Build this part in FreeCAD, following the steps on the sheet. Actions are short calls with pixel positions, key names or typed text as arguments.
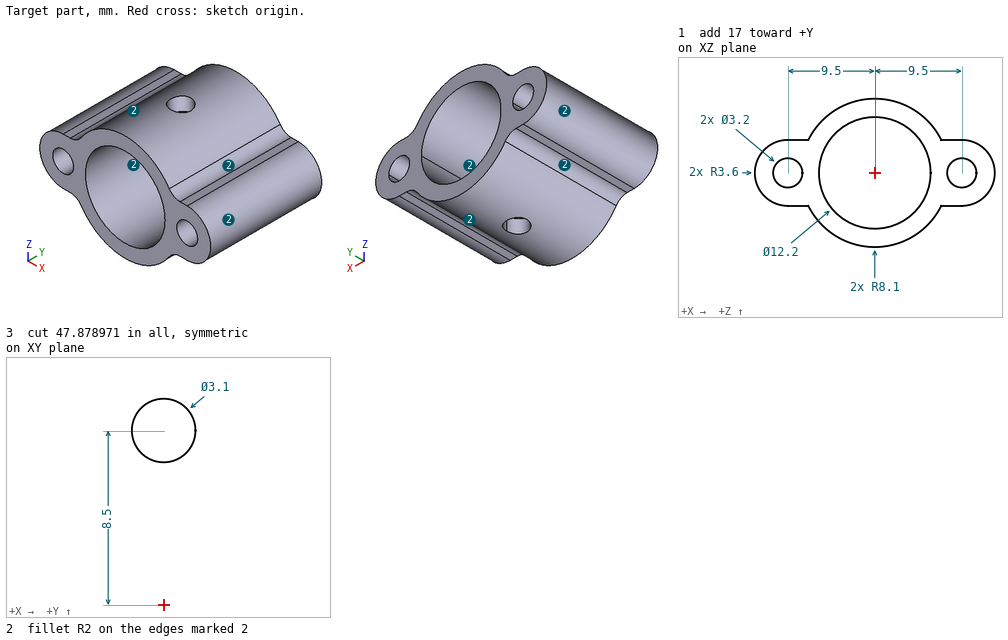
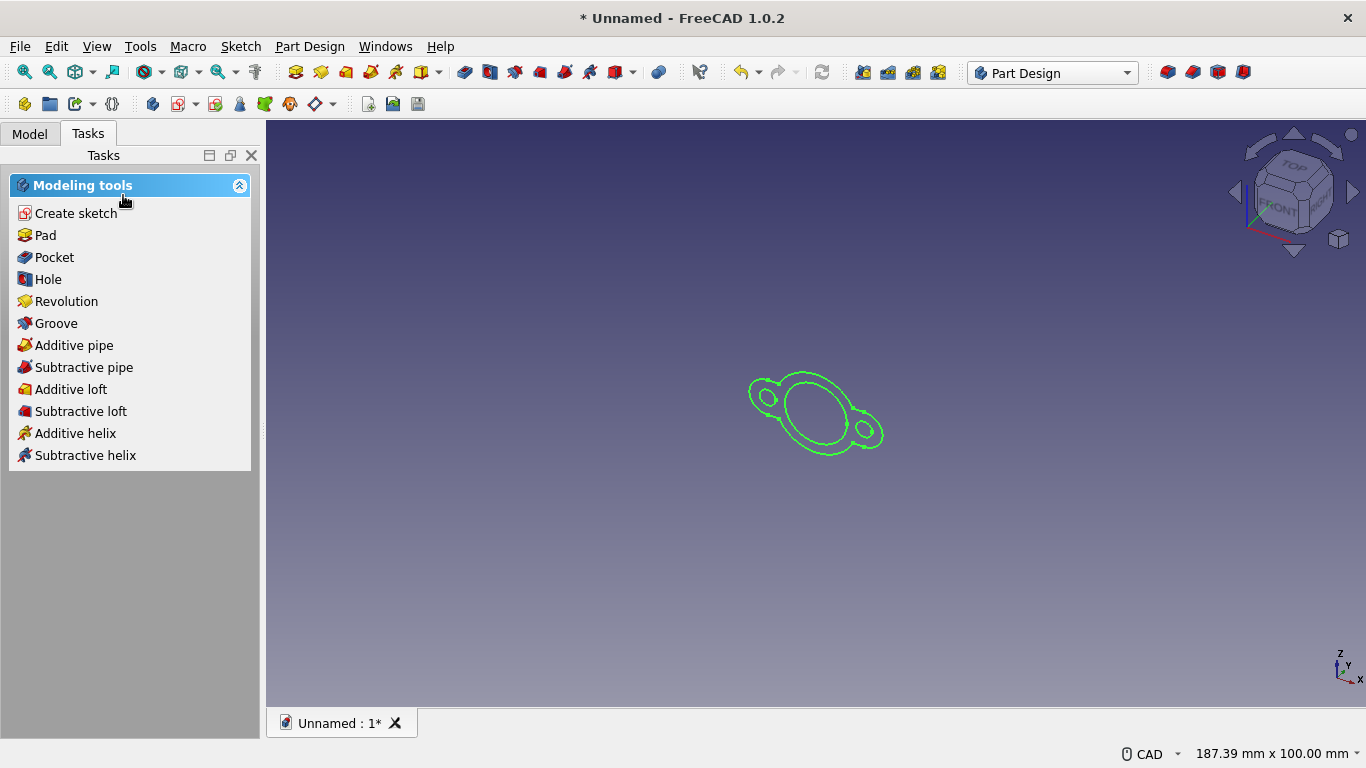
click(296, 72)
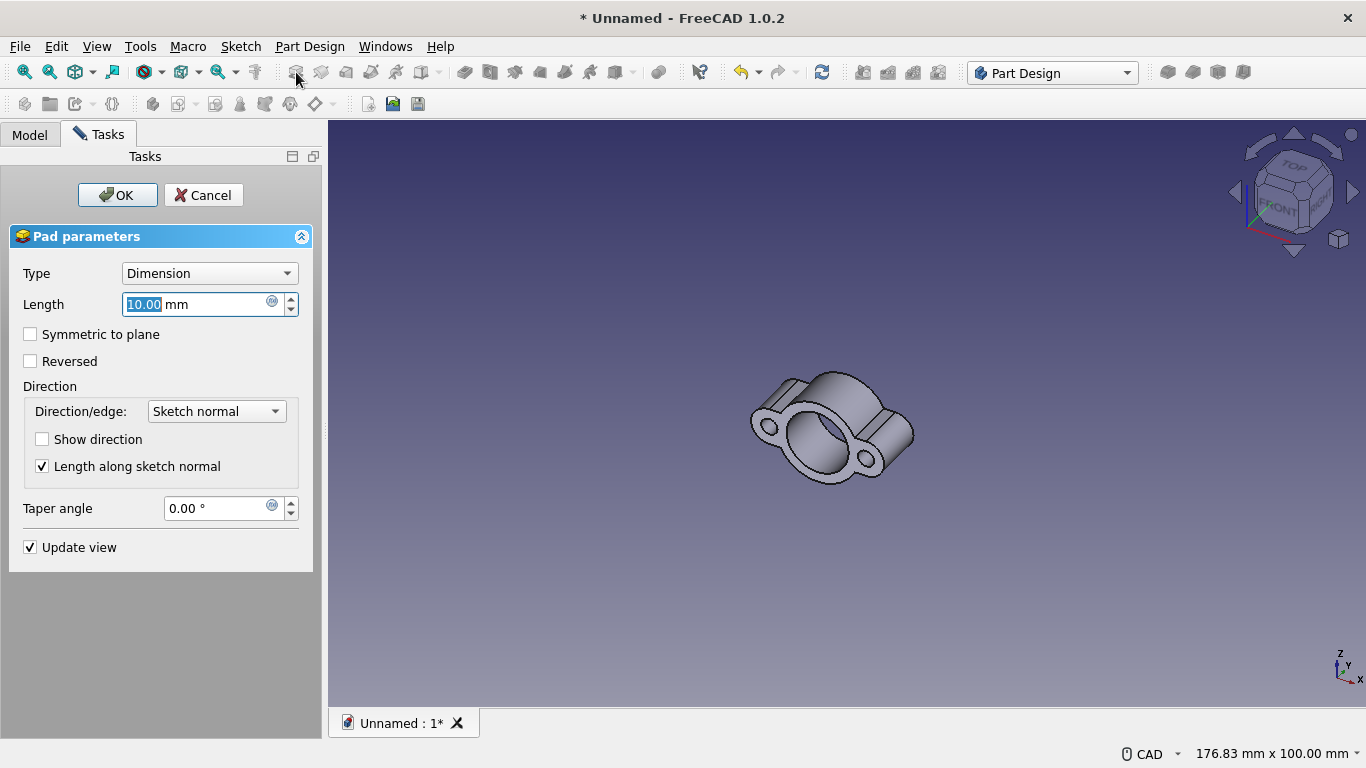
text(17)
key(Tab)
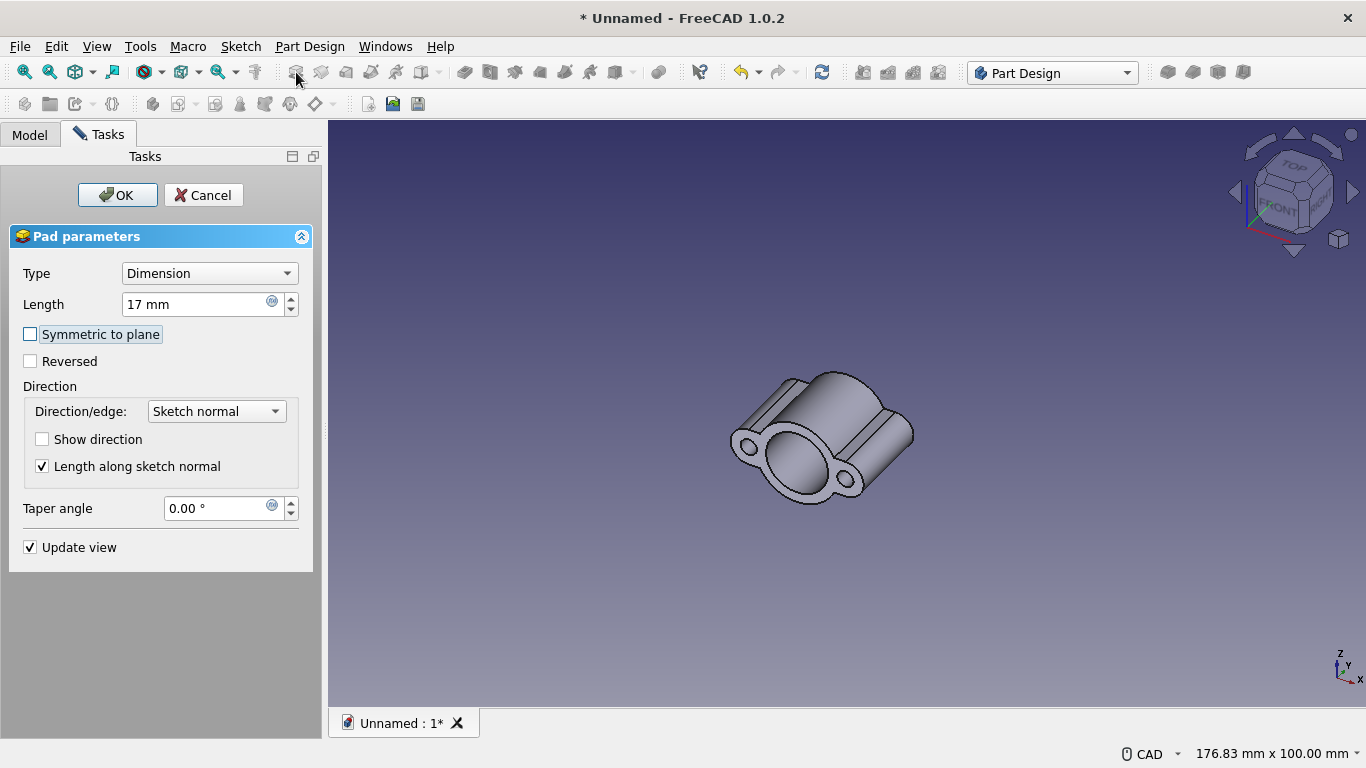
click(31, 361)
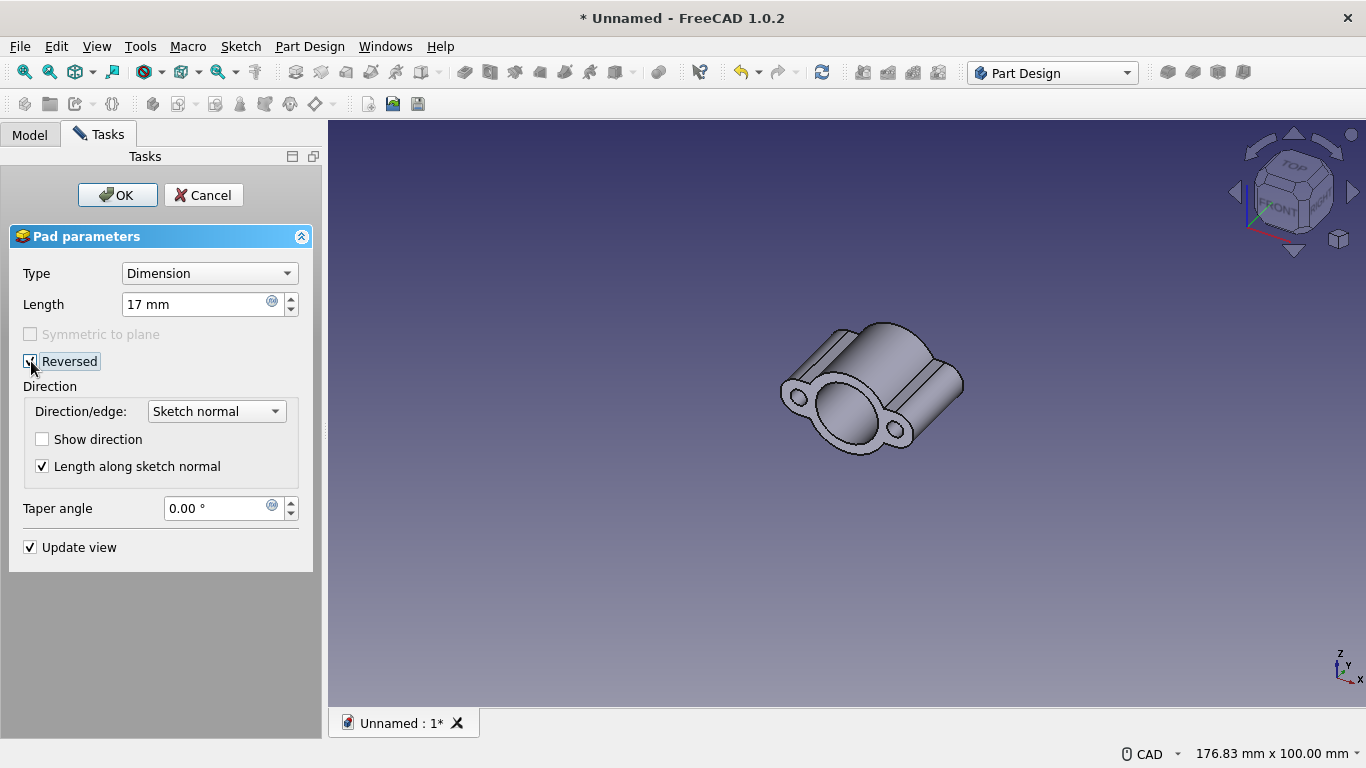
click(118, 195)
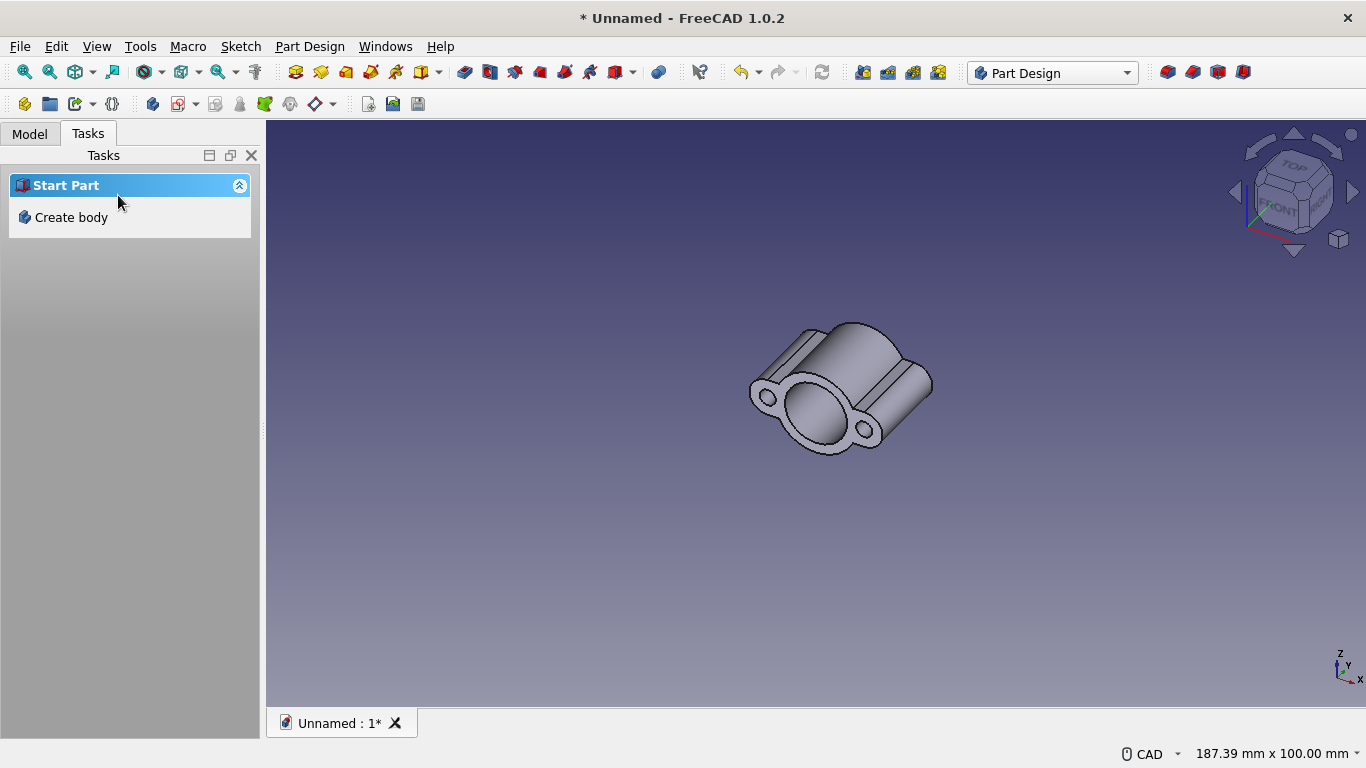
key(v)
key(f)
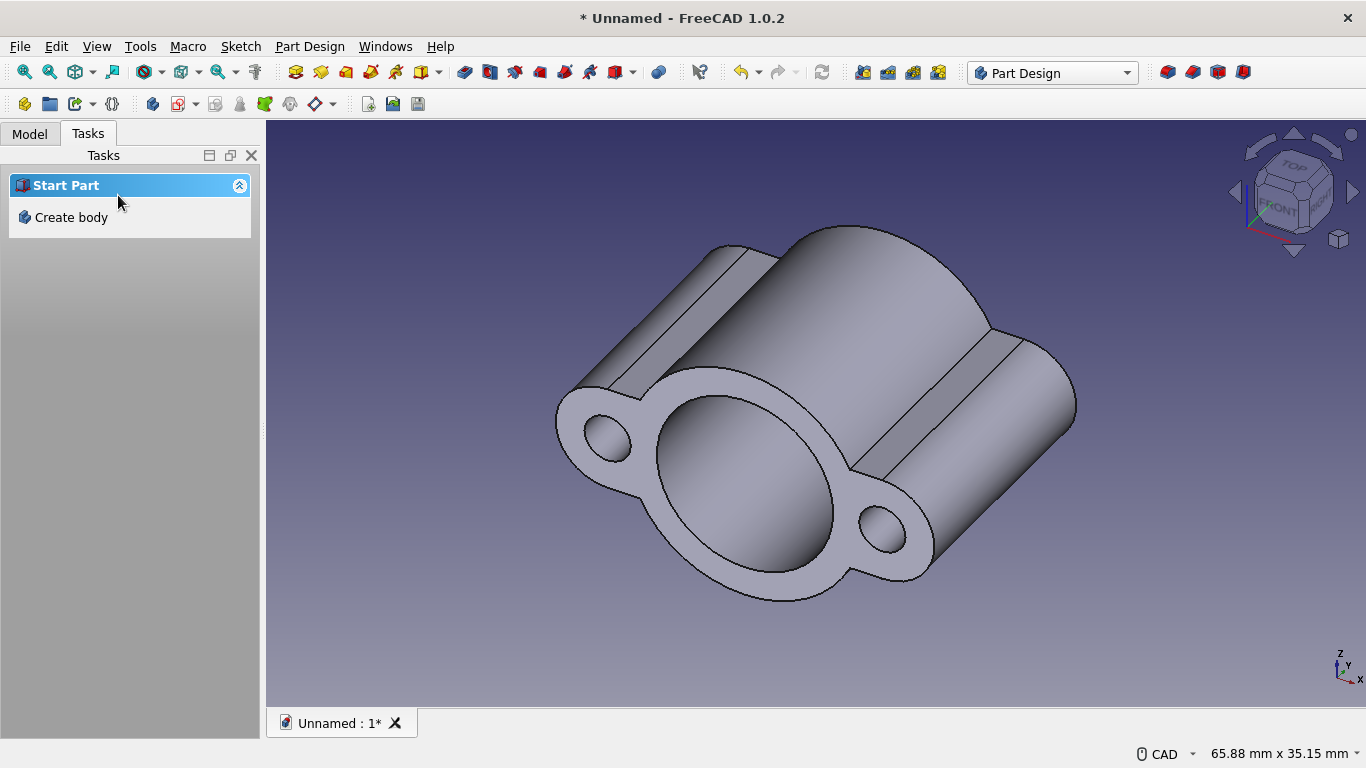
key(0)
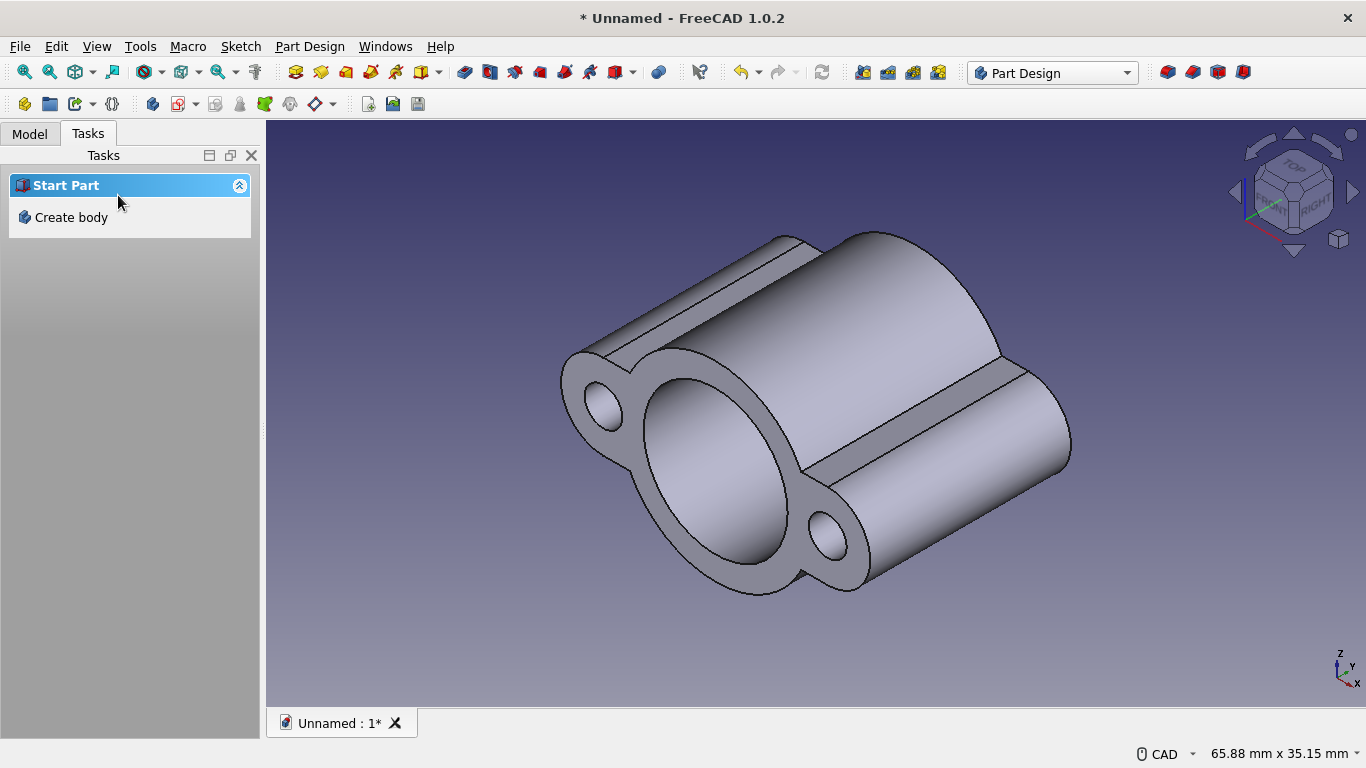
key(2)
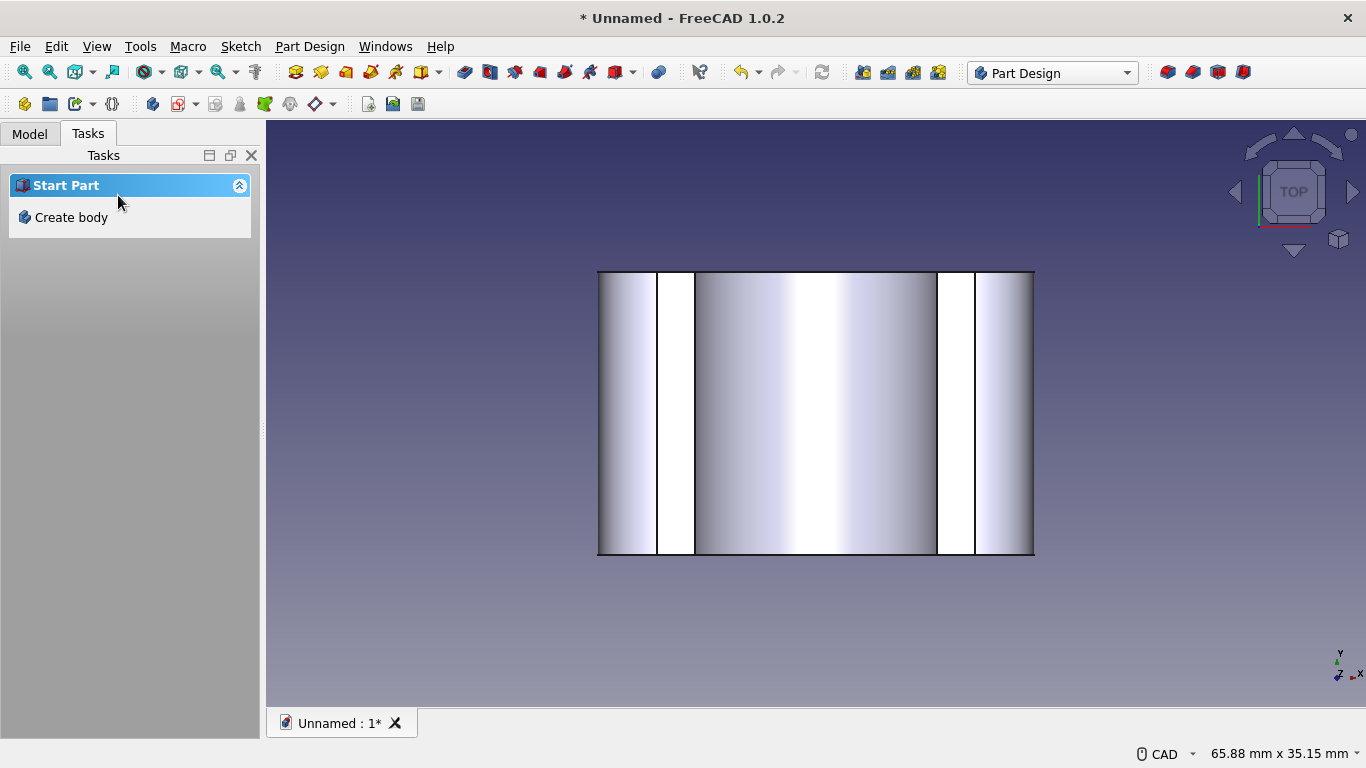
key(1)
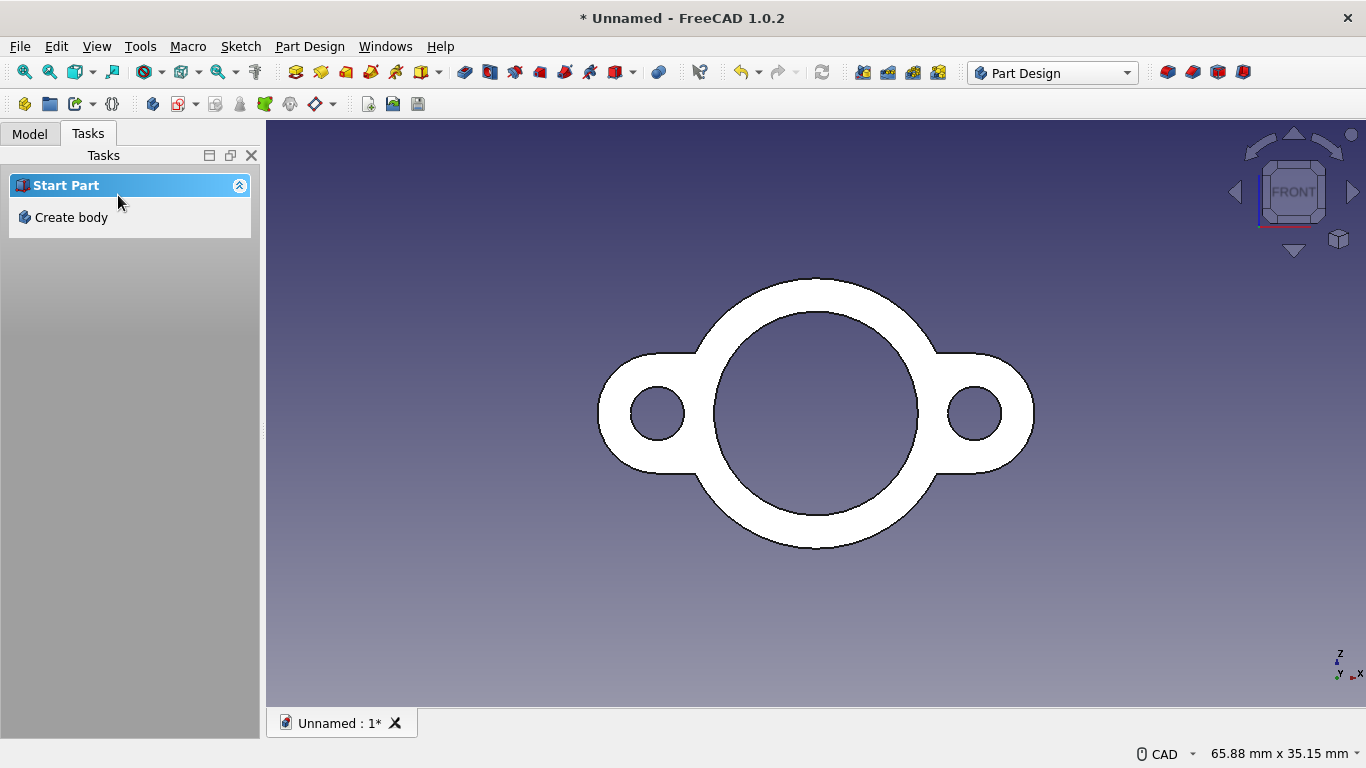
key(3)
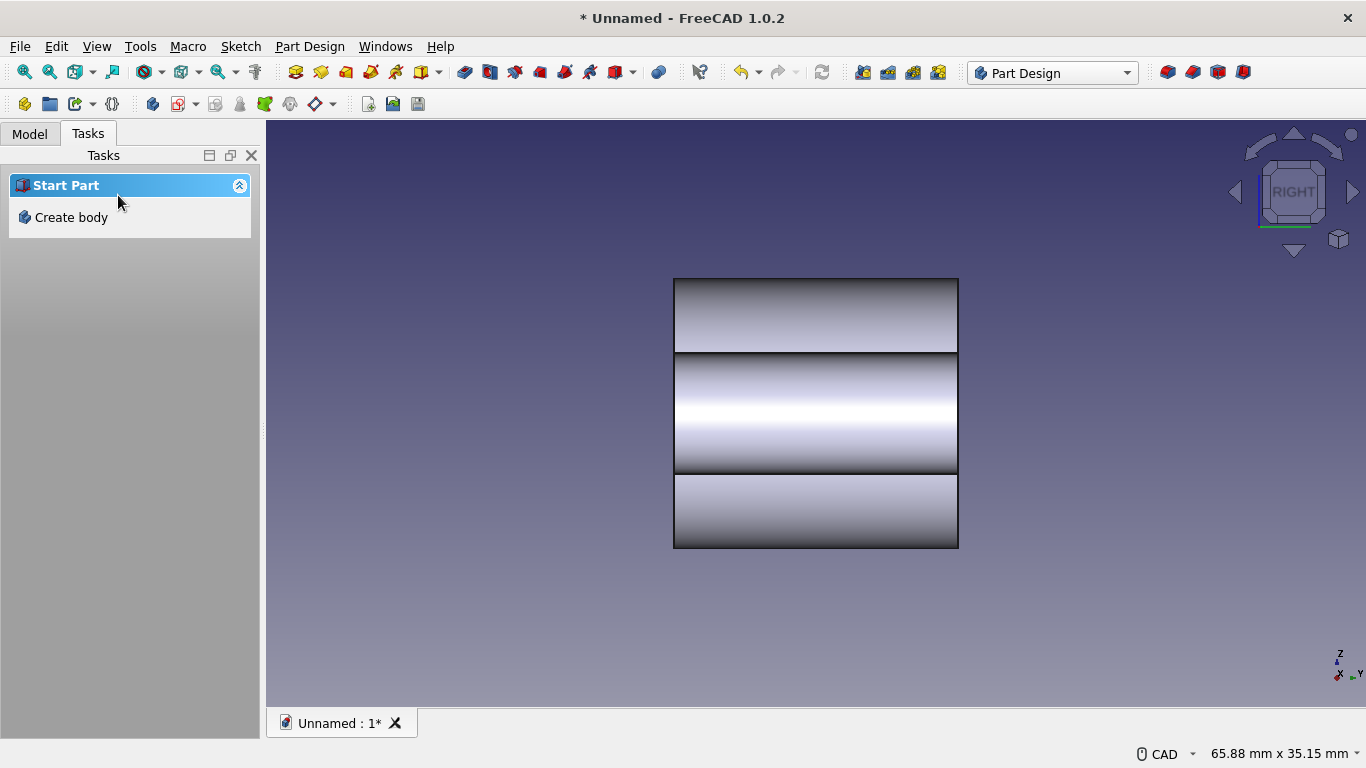
key(5)